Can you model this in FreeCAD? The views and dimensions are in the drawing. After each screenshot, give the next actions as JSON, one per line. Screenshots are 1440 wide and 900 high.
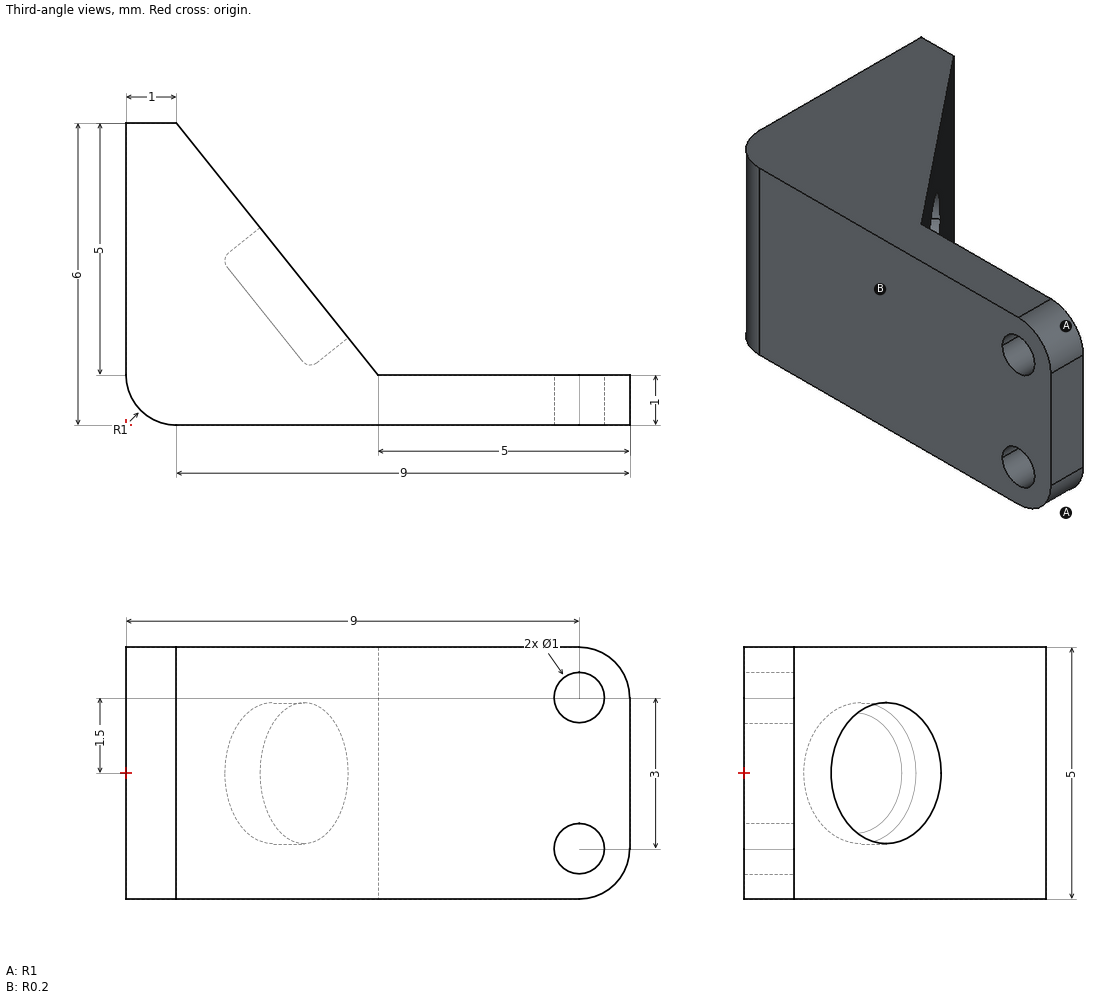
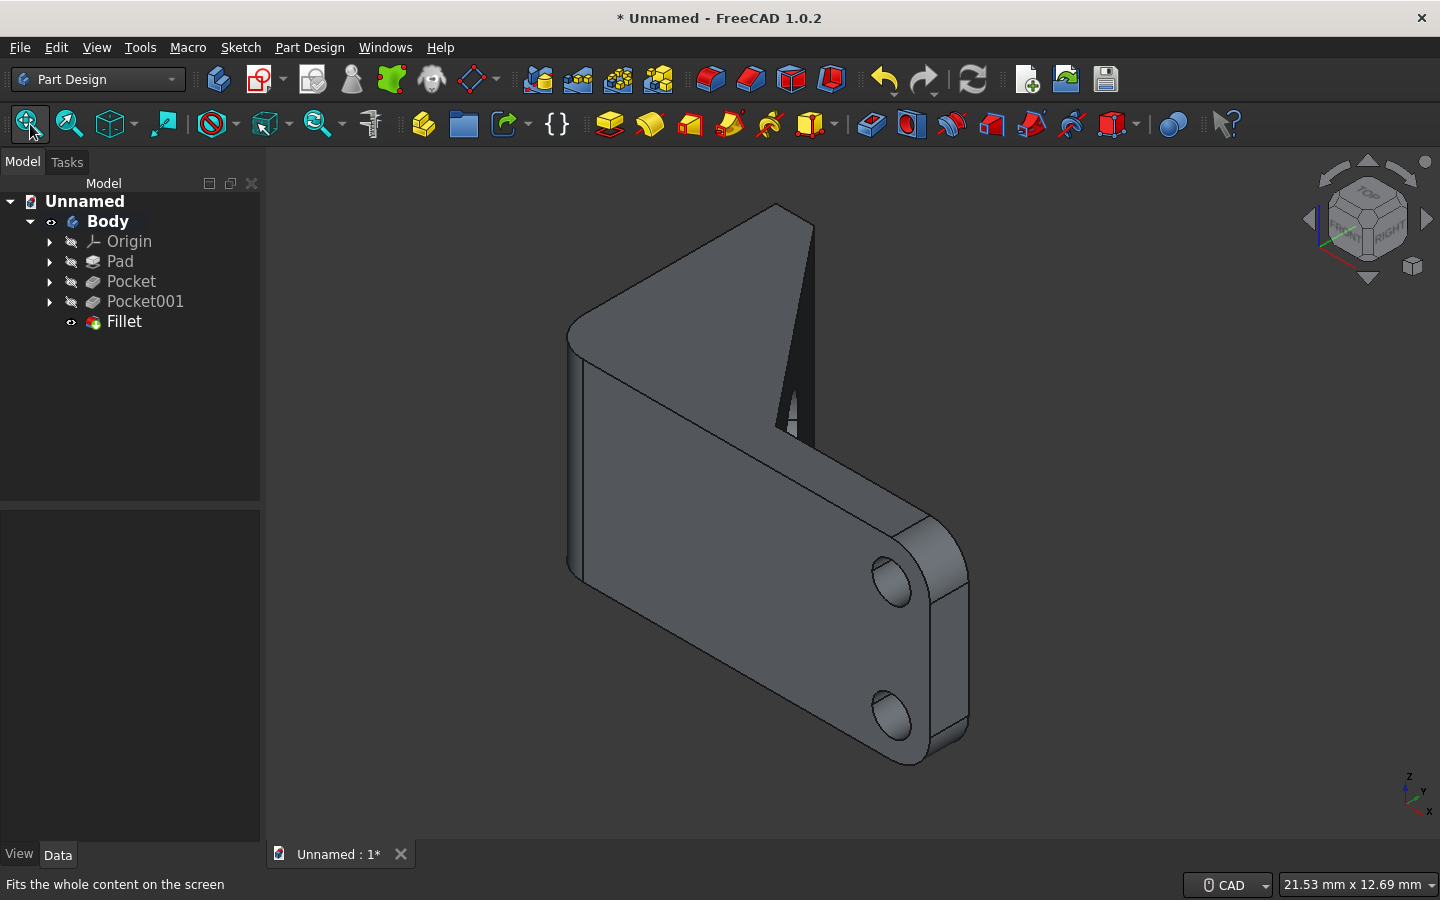
{"action": "key", "text": "2"}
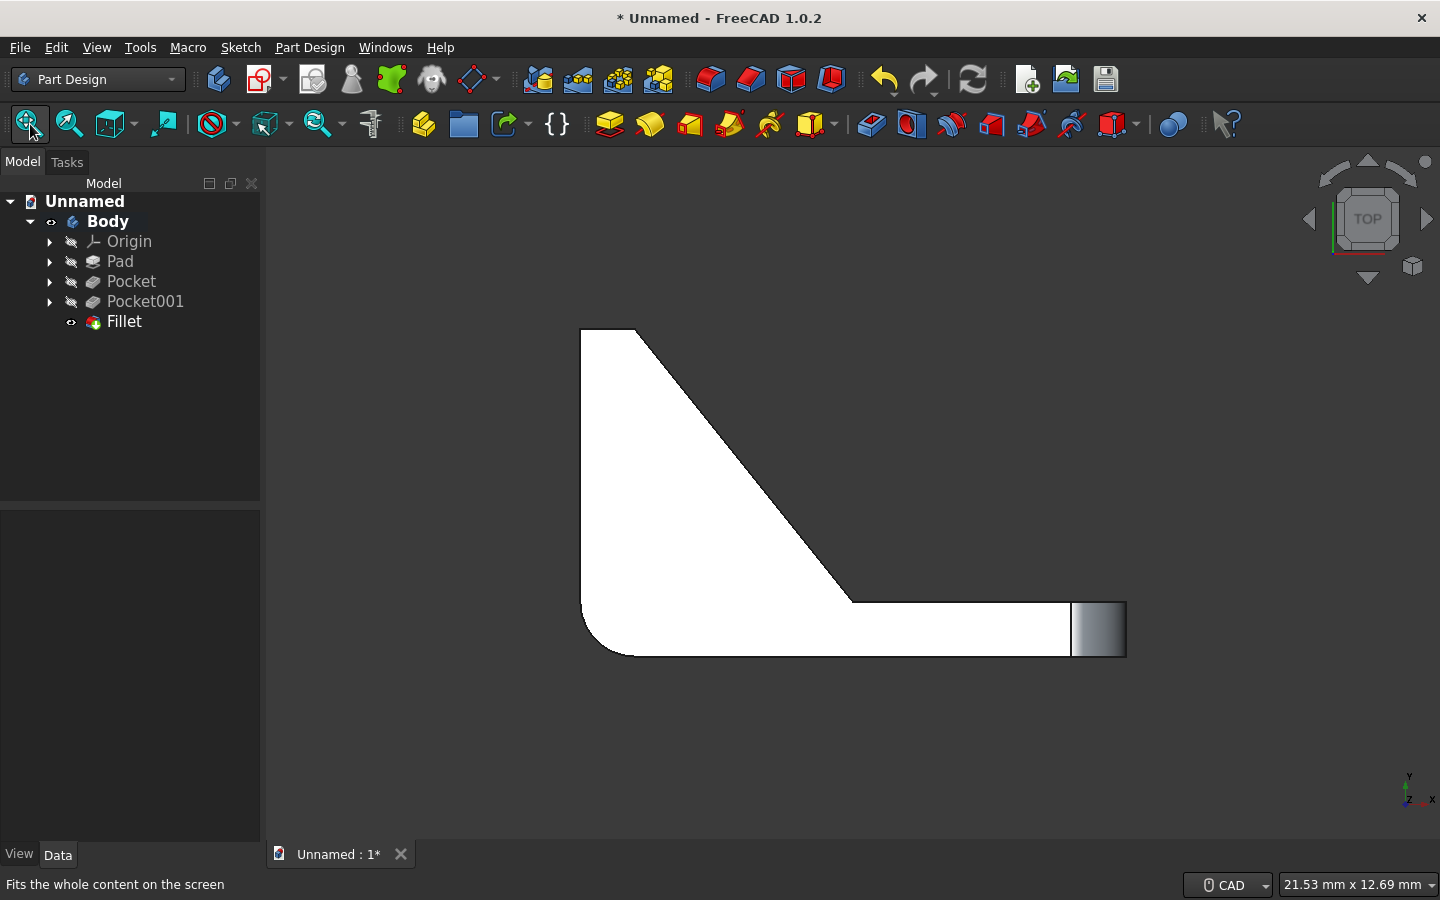
{"action": "key", "text": "1"}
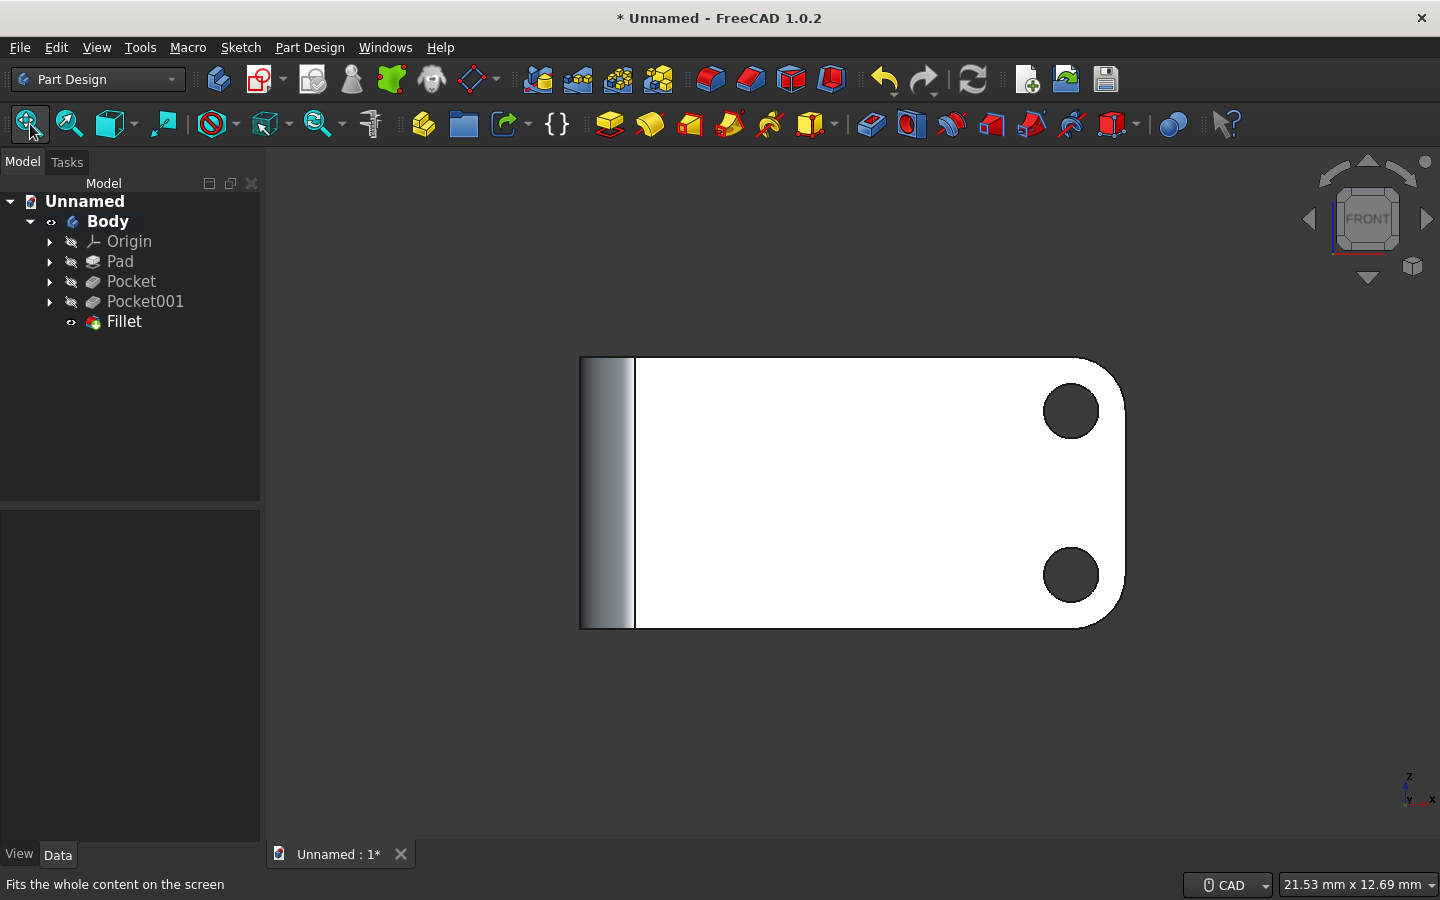
{"action": "key", "text": "3"}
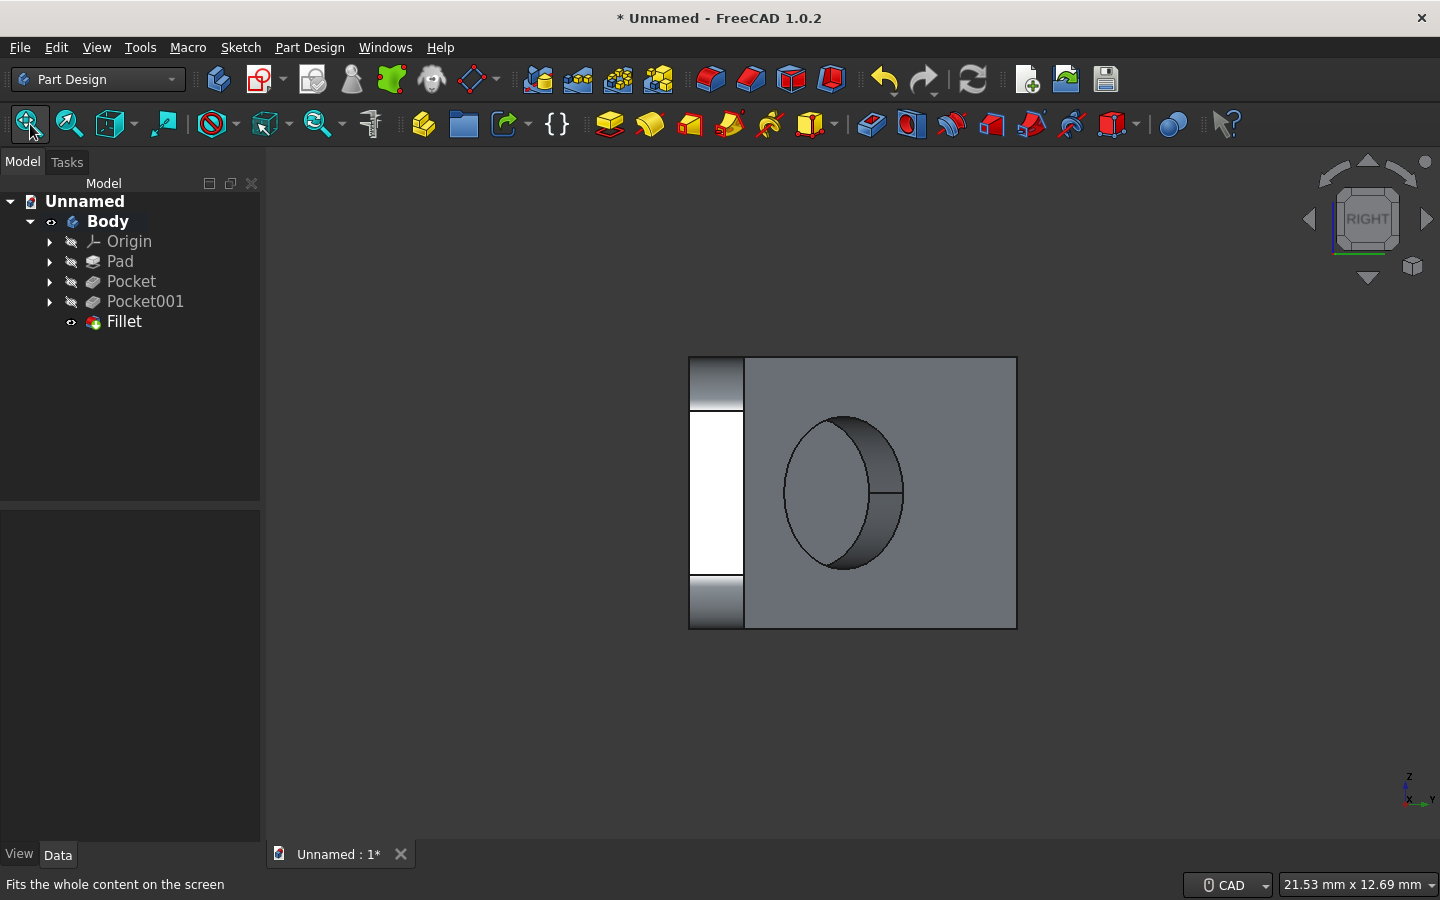
{"action": "left_click", "coordinate": [30, 124]}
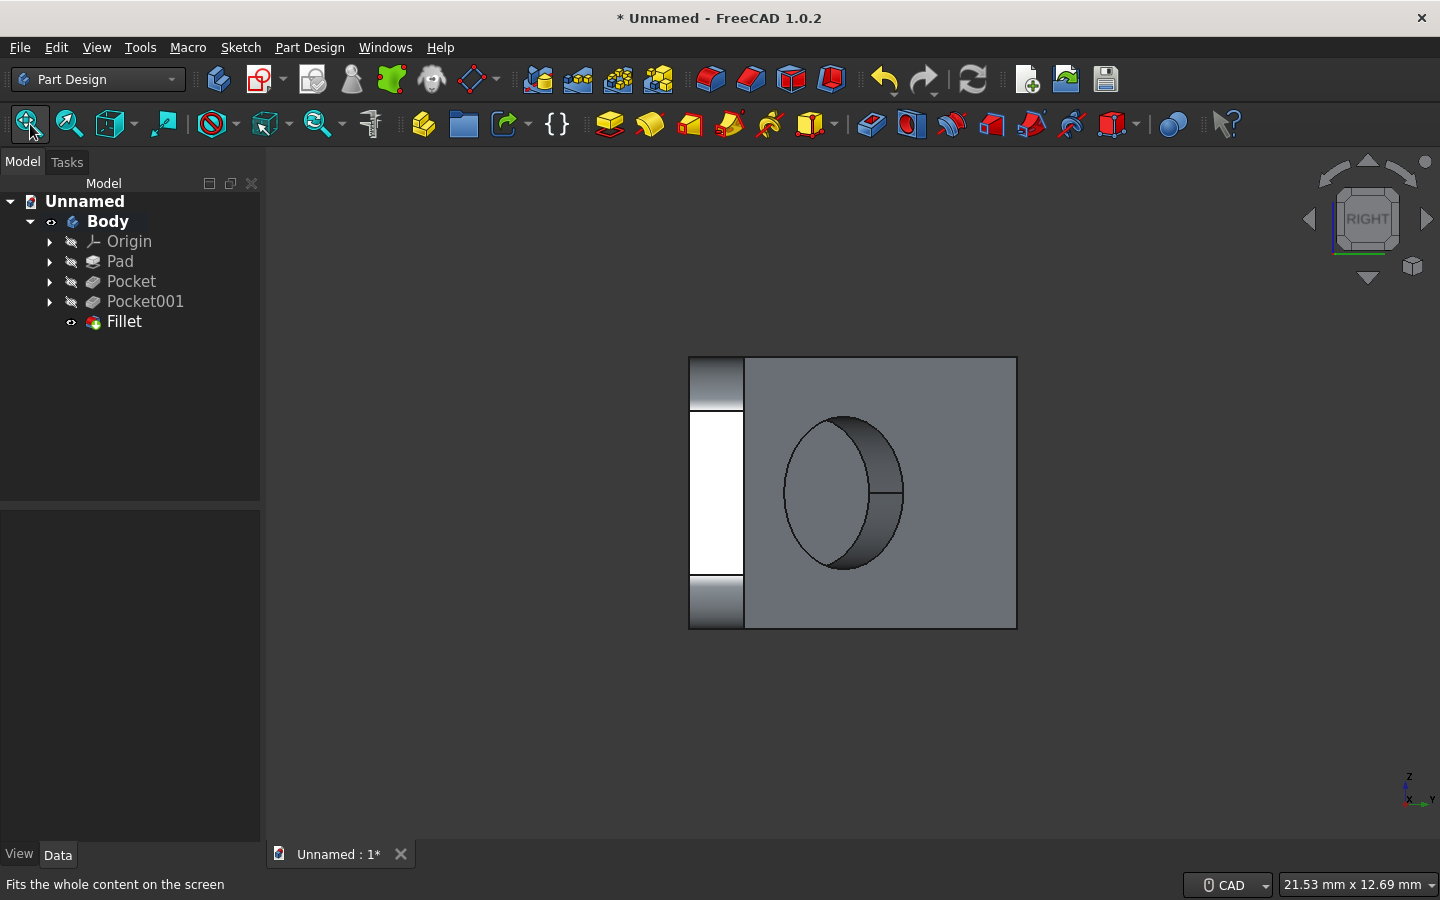
{"action": "key", "text": "5"}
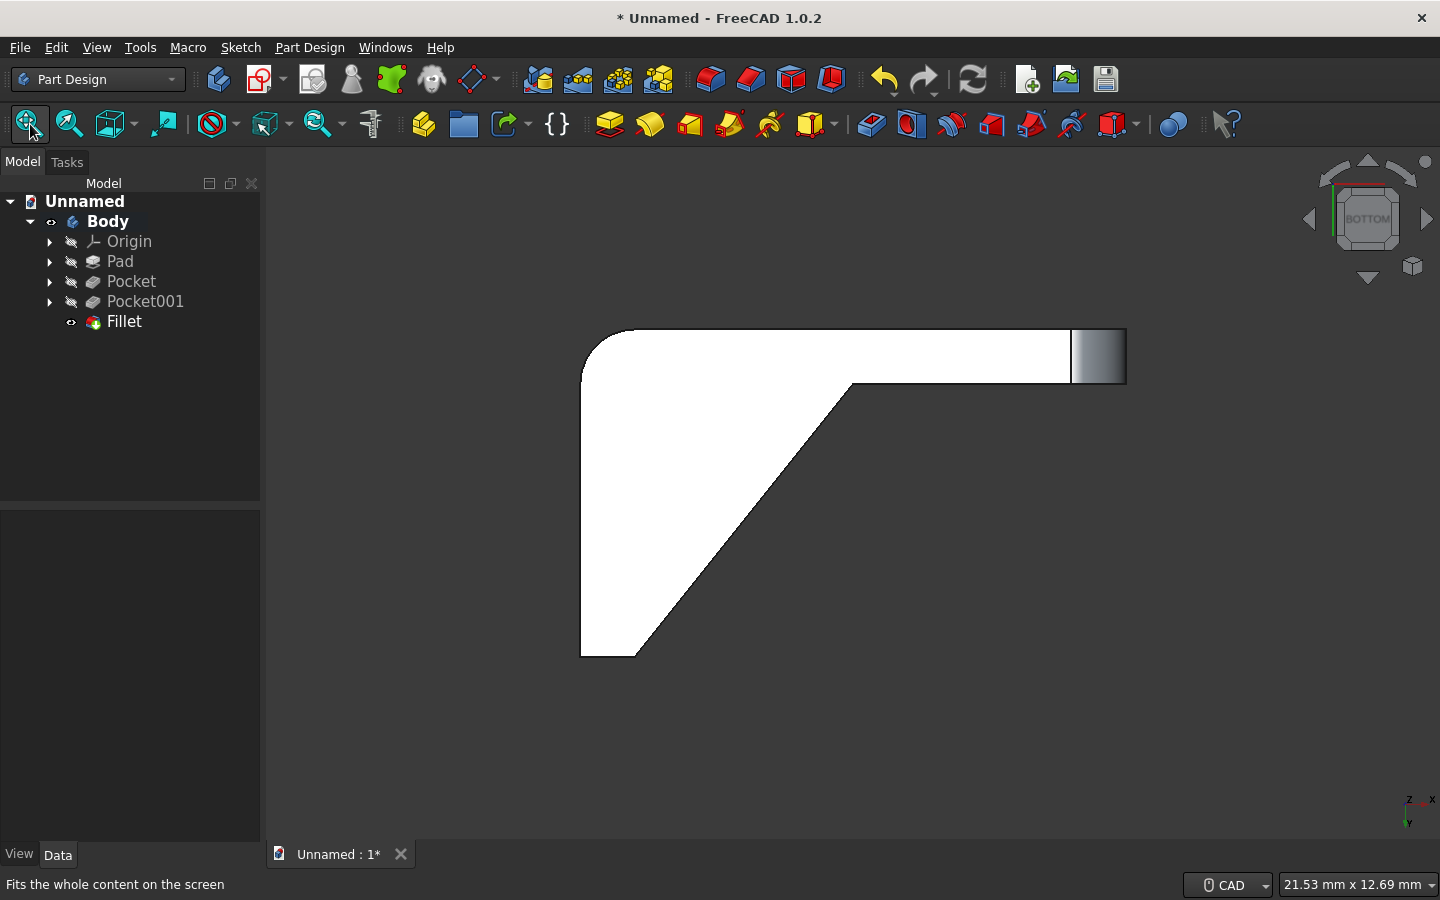
{"action": "key", "text": "4"}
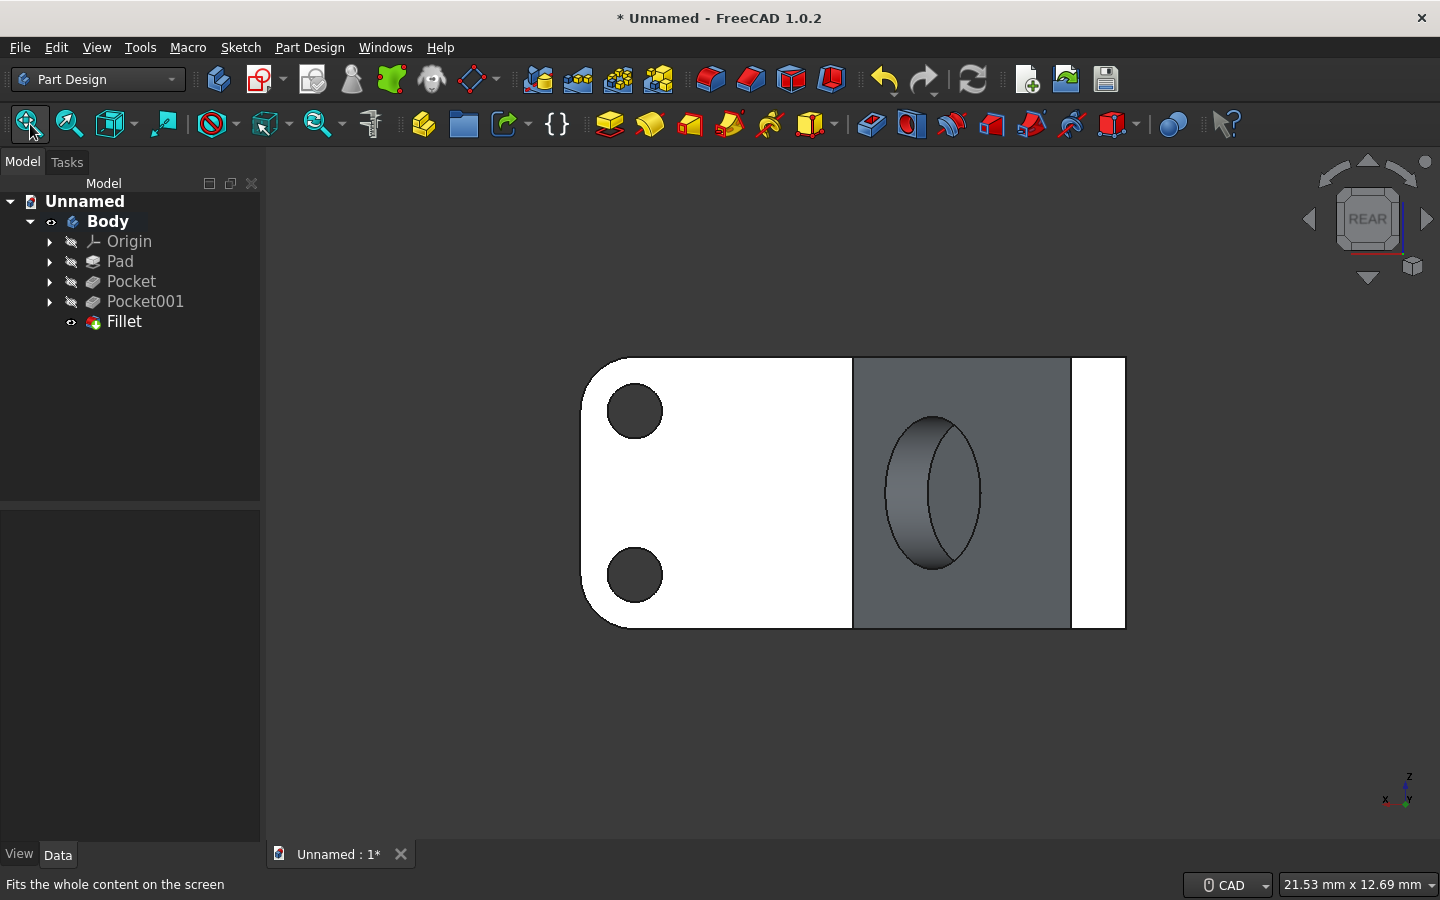
{"action": "key", "text": "6"}